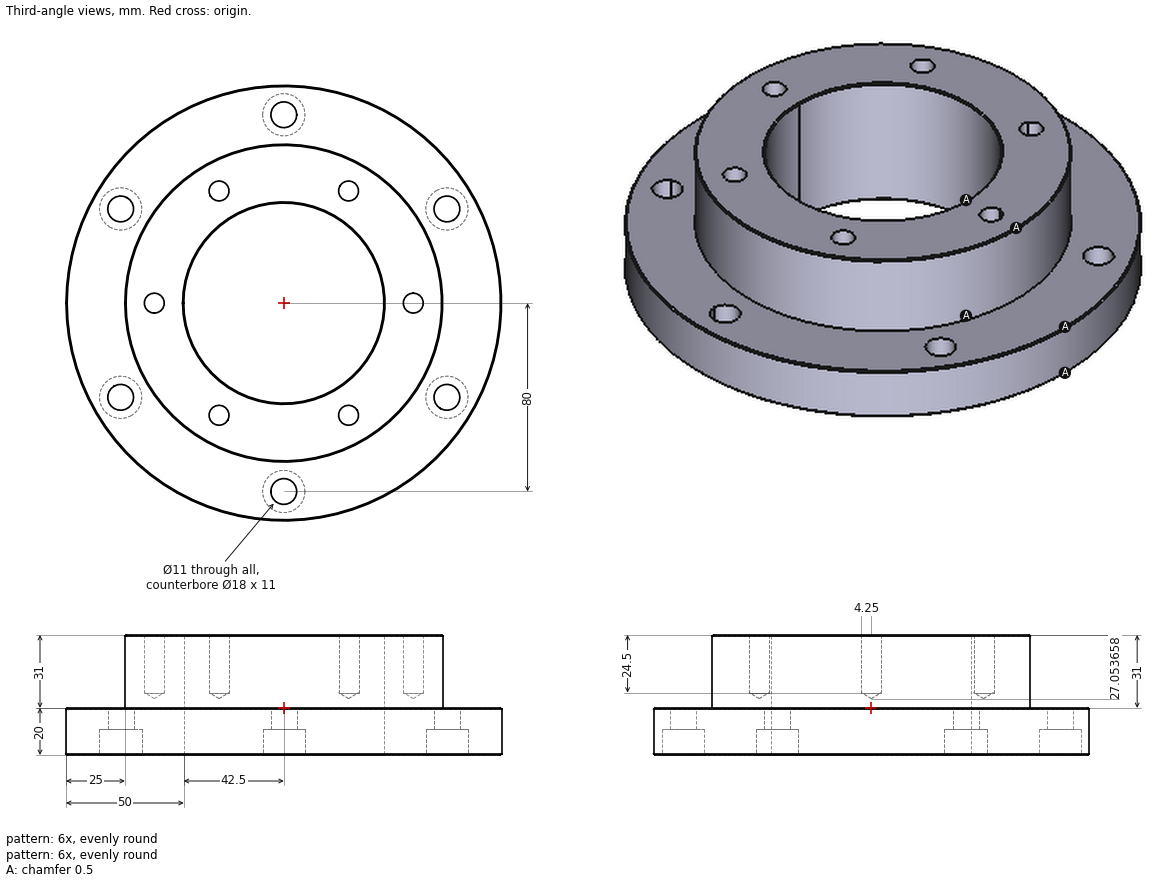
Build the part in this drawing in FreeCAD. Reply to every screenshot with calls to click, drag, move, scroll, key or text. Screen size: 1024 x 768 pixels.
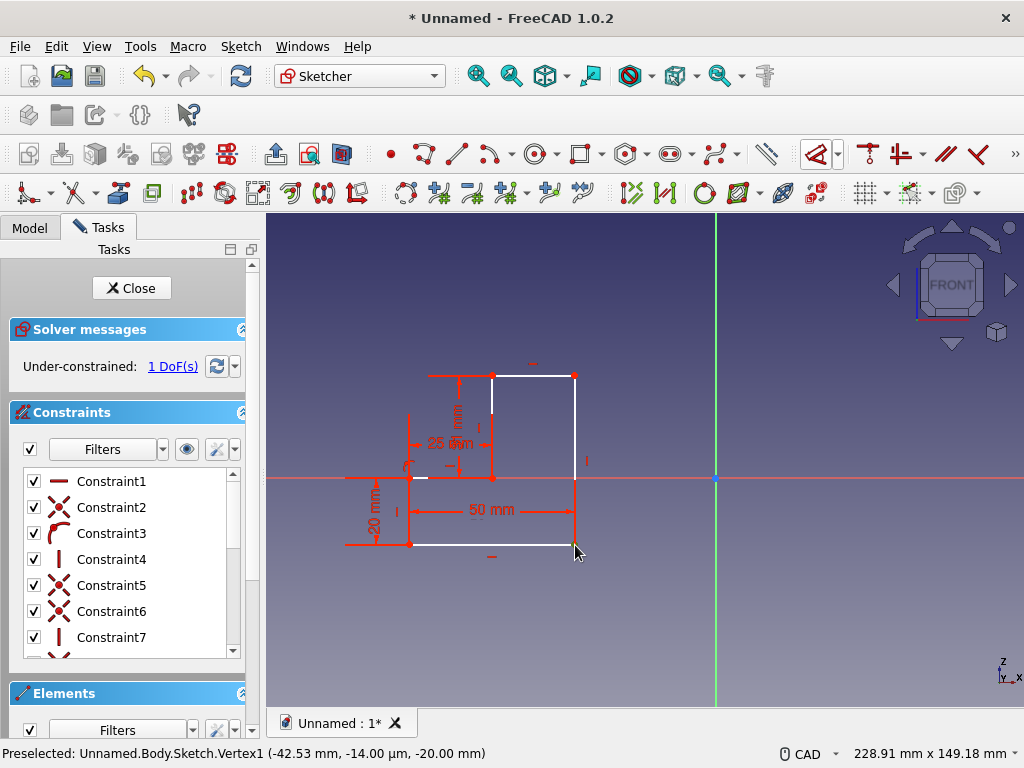
click(838, 154)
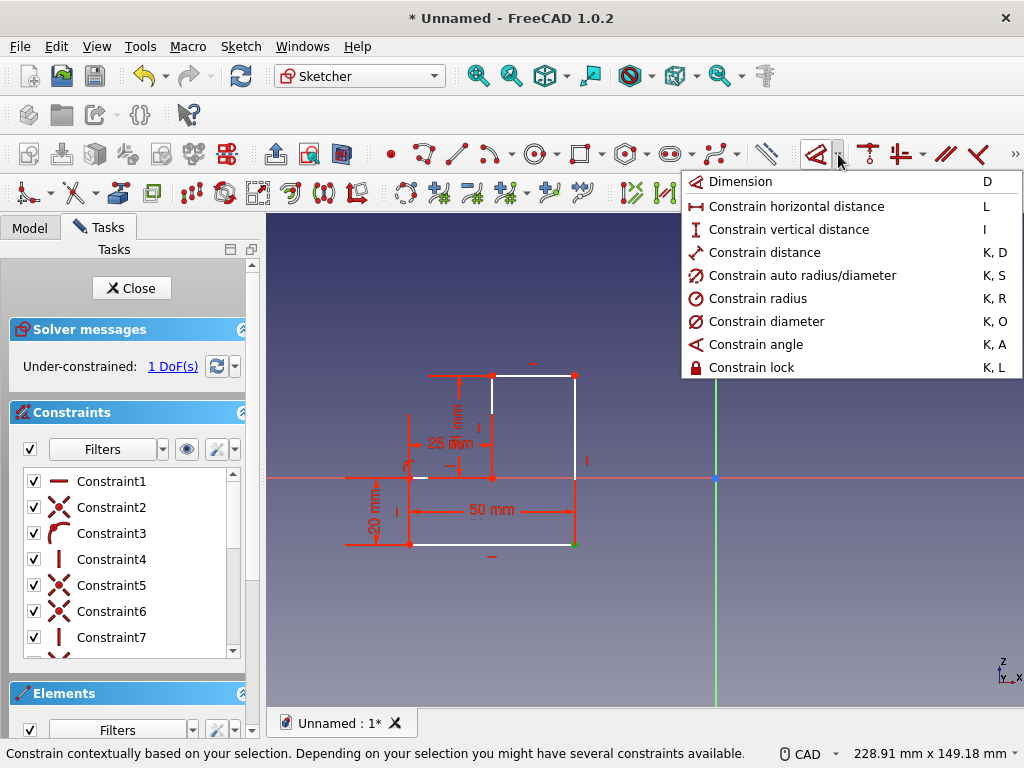
click(852, 206)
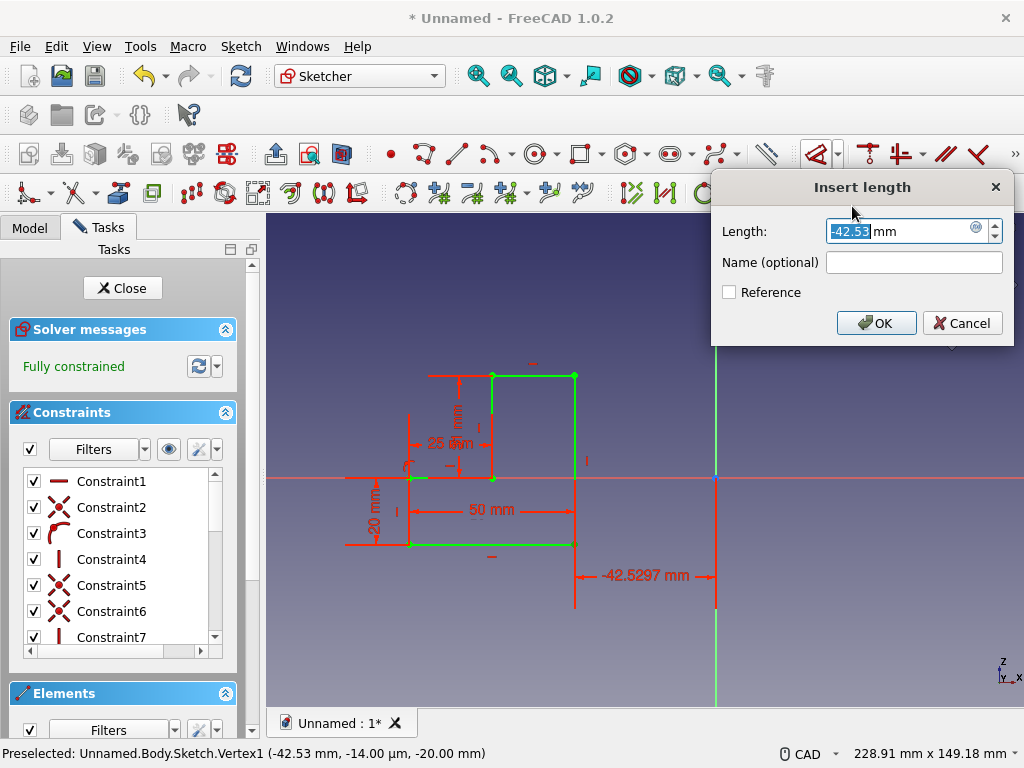
text(-42.5)
key(Return)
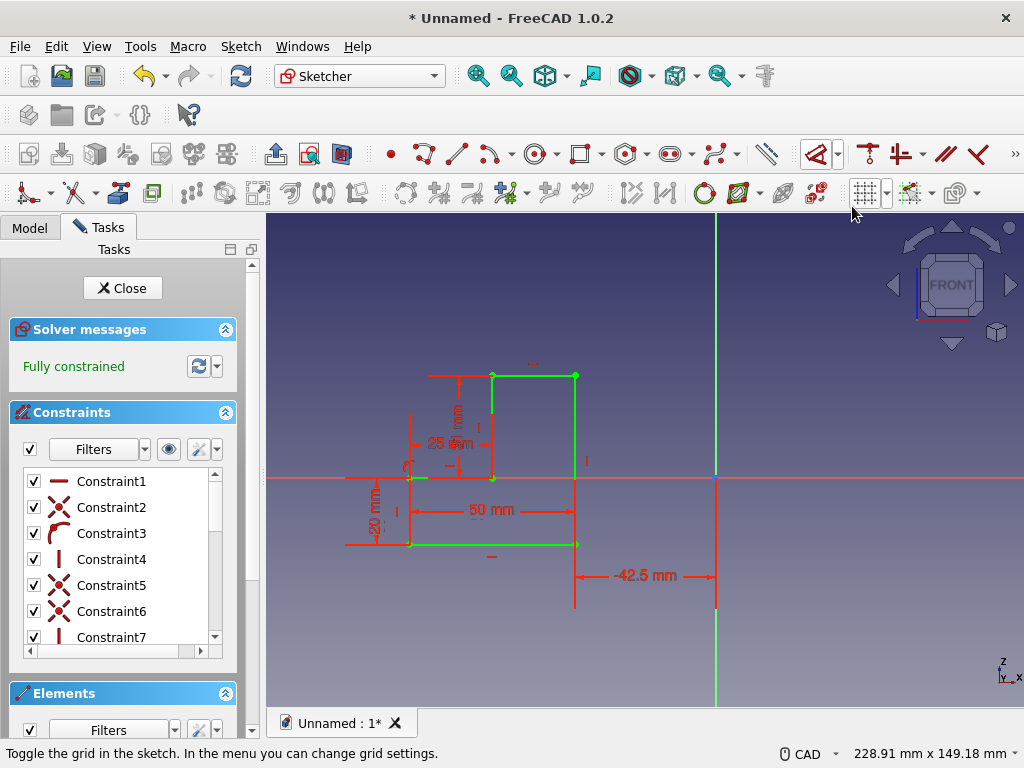
click(123, 288)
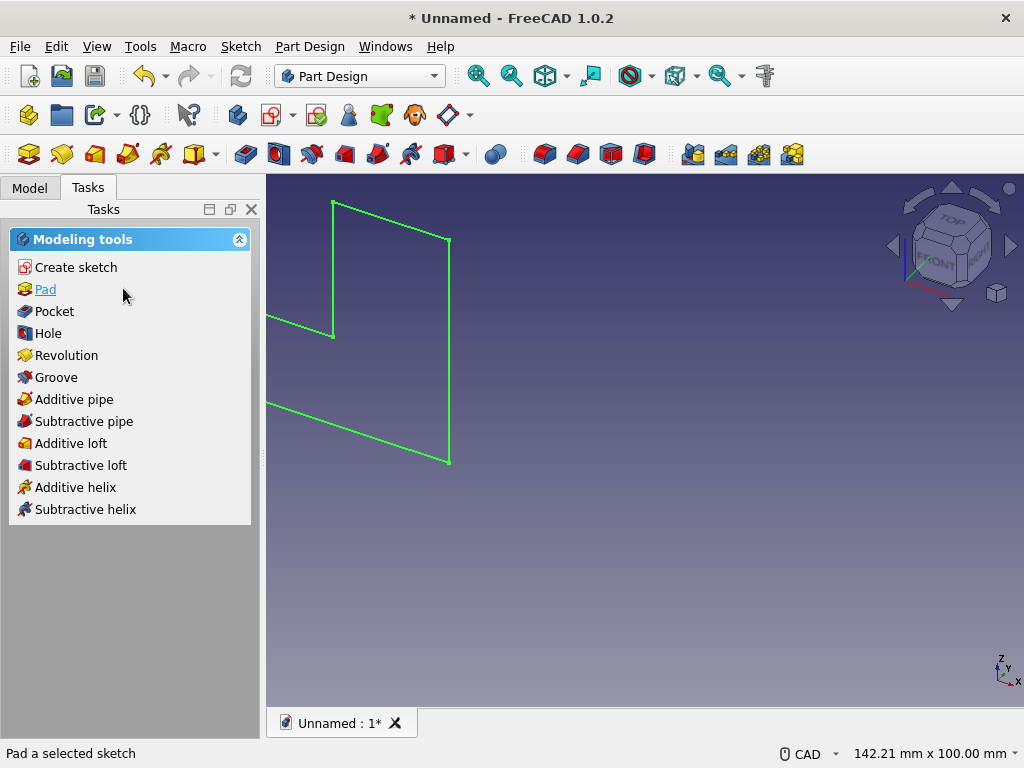
click(62, 154)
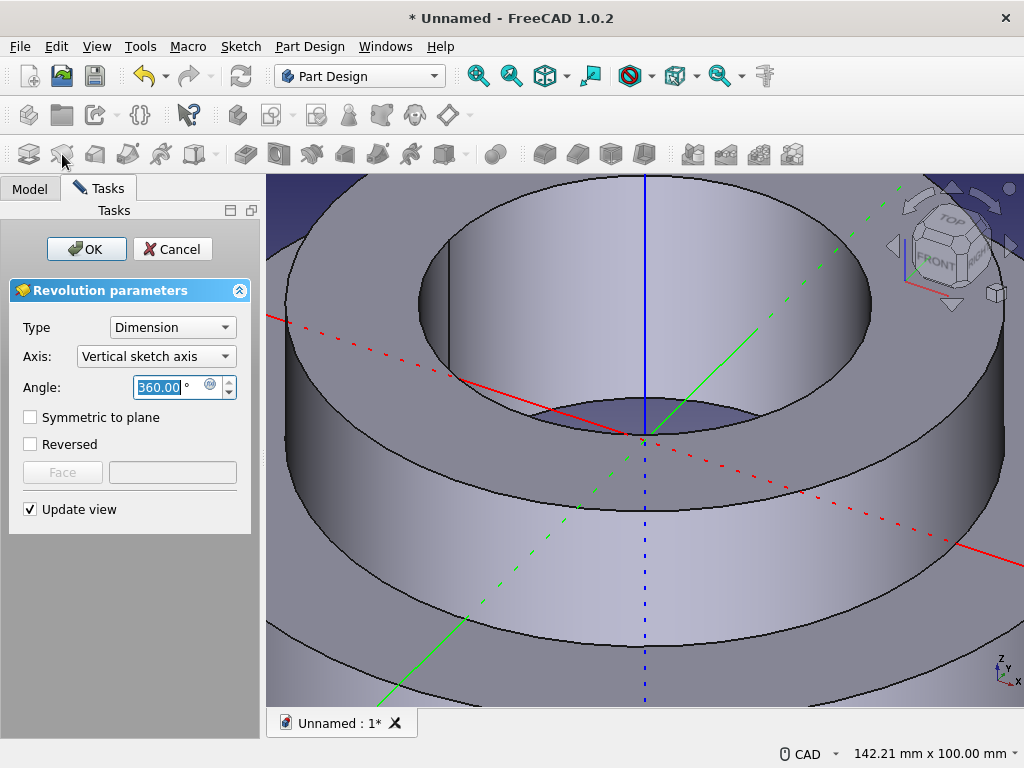
click(87, 249)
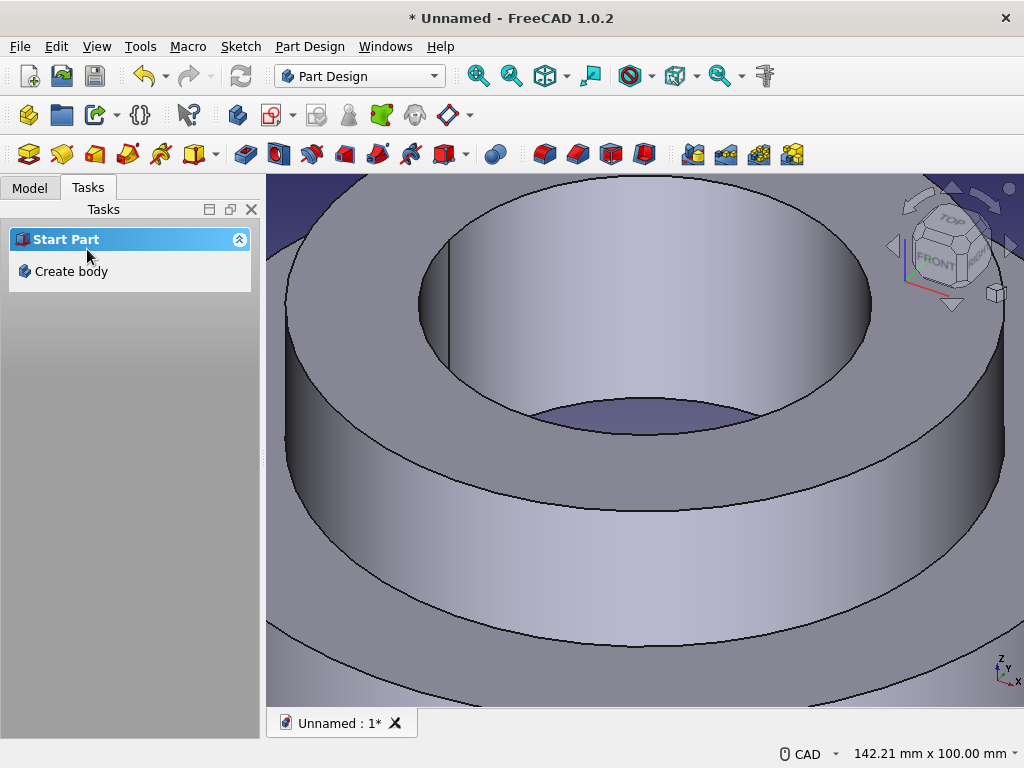
click(479, 76)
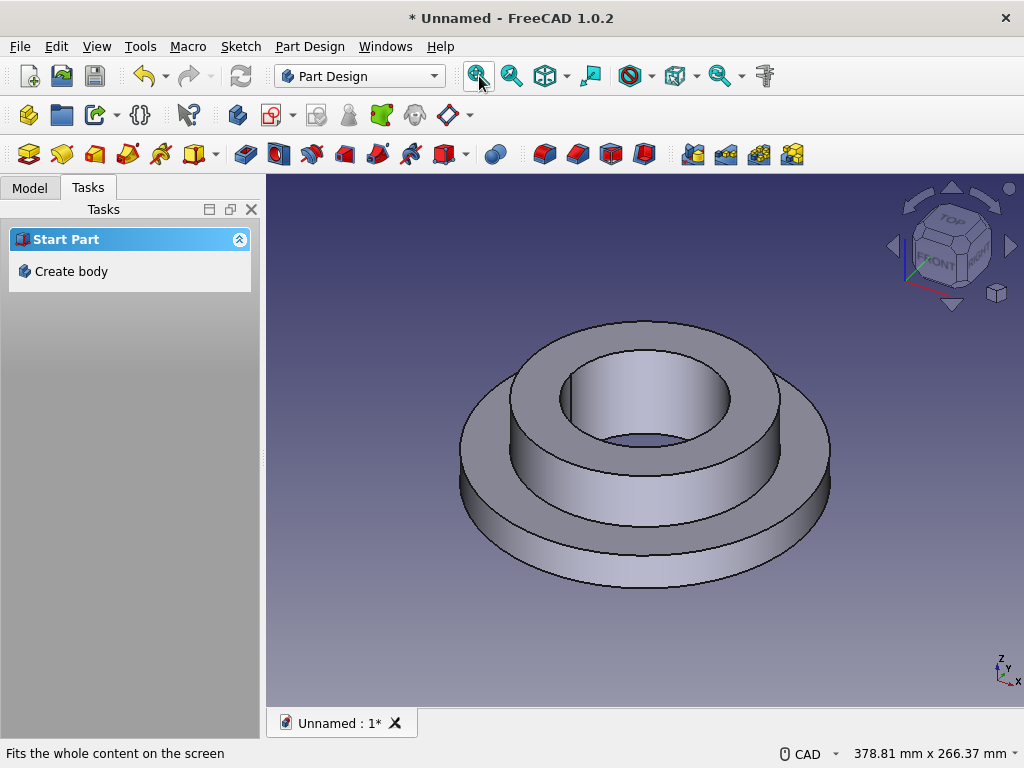
key(5)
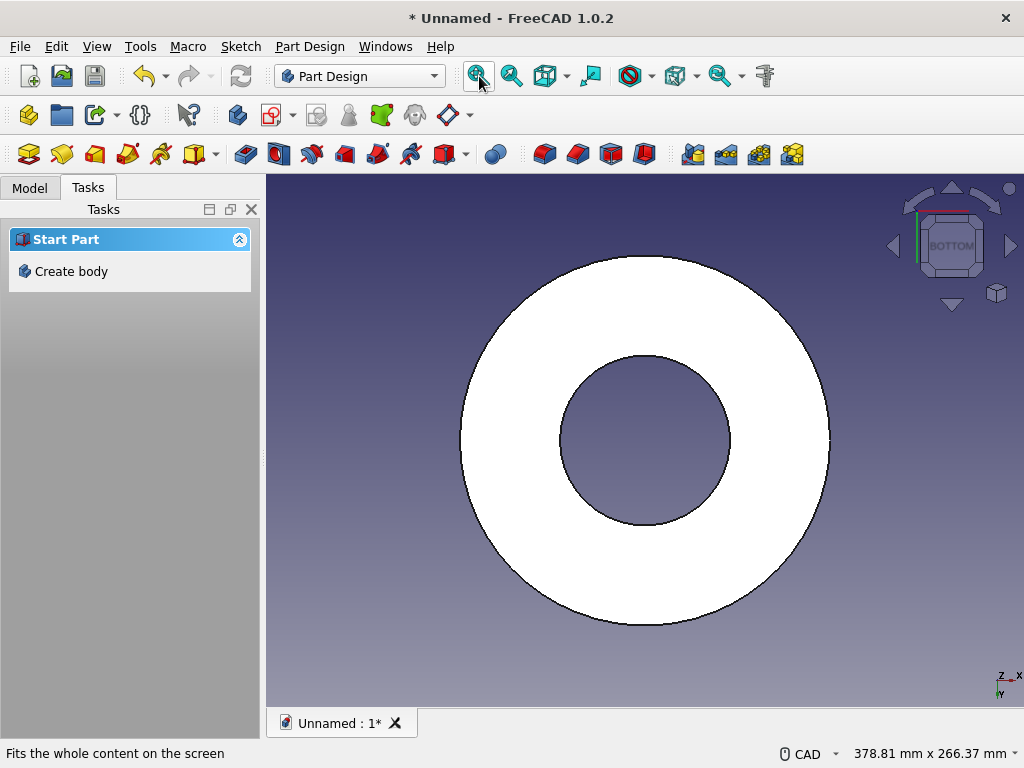
click(751, 545)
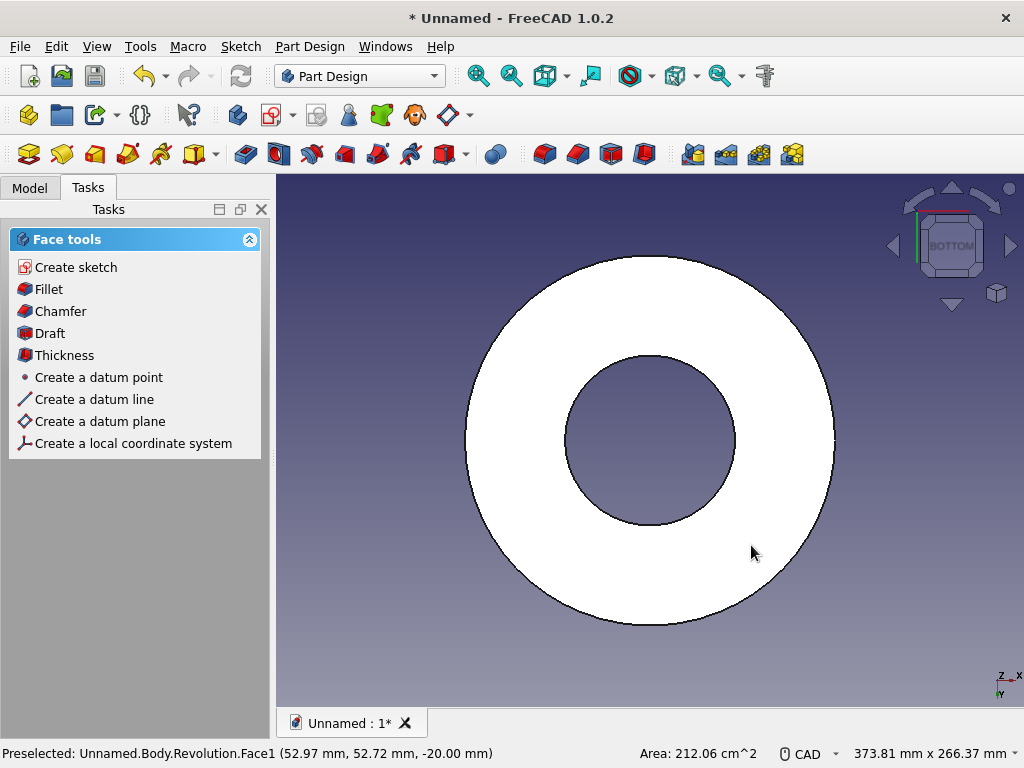
click(270, 116)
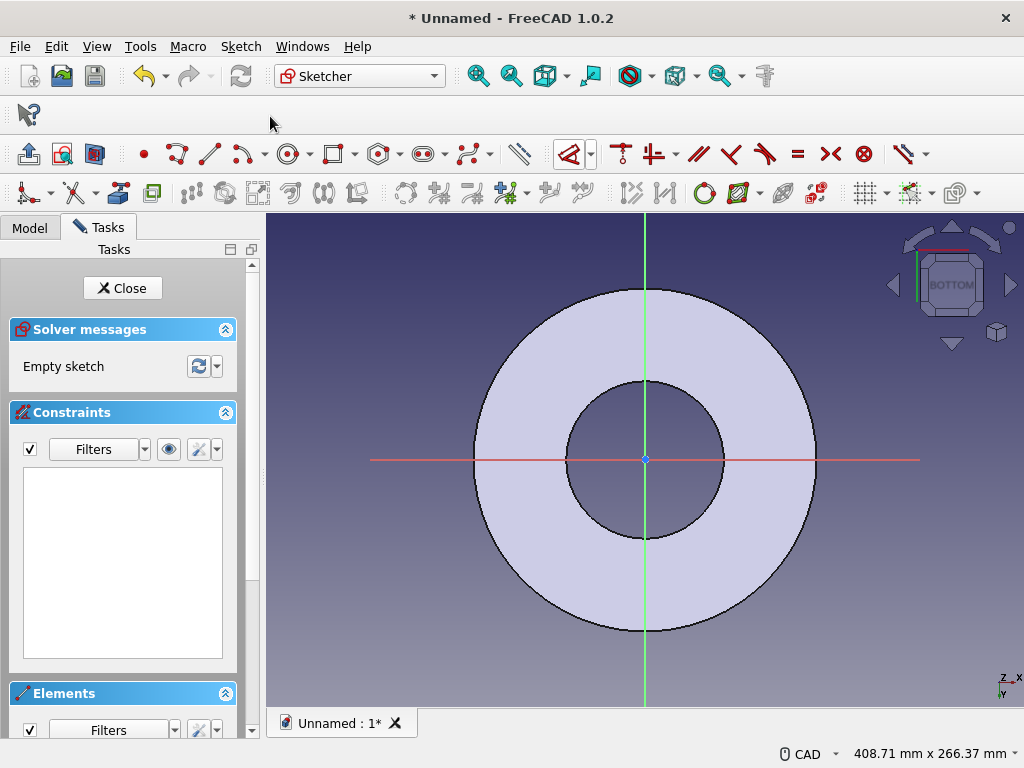
scroll(649, 302, up, 14)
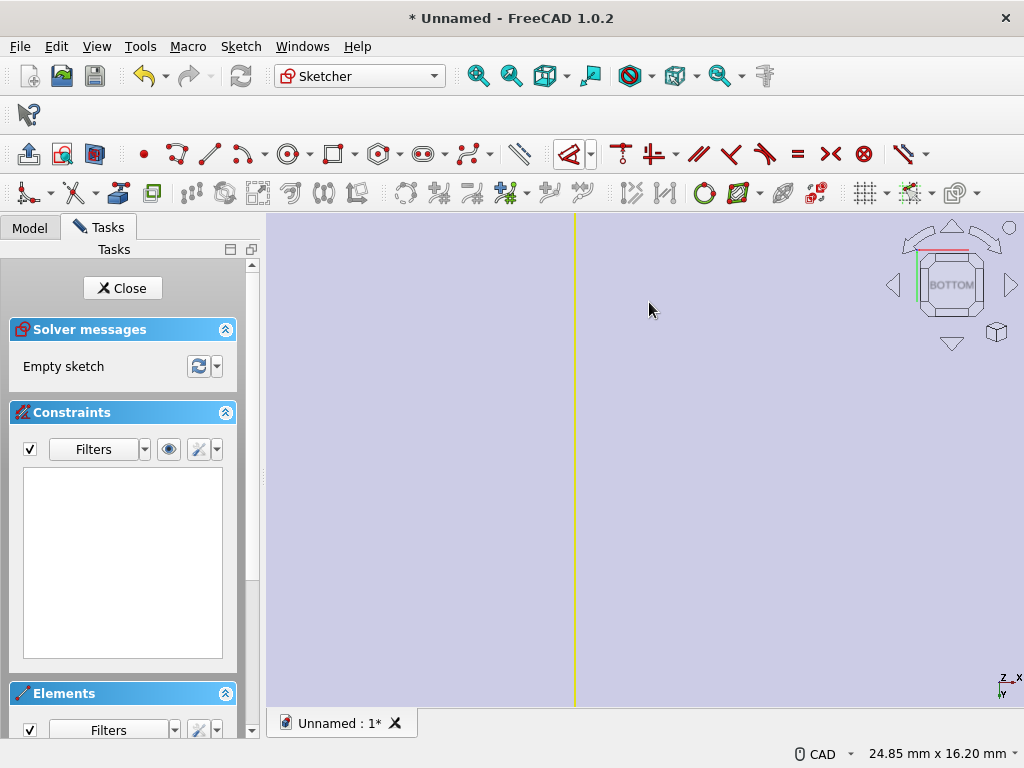
key(g)
key(c)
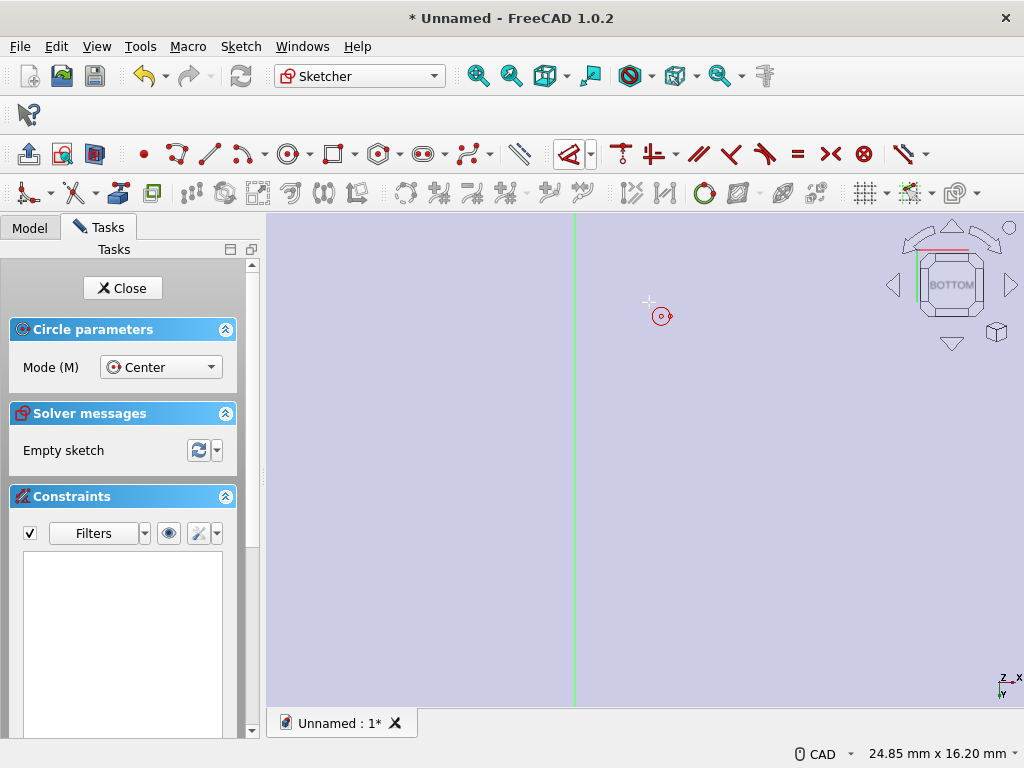
click(575, 458)
move(694, 339)